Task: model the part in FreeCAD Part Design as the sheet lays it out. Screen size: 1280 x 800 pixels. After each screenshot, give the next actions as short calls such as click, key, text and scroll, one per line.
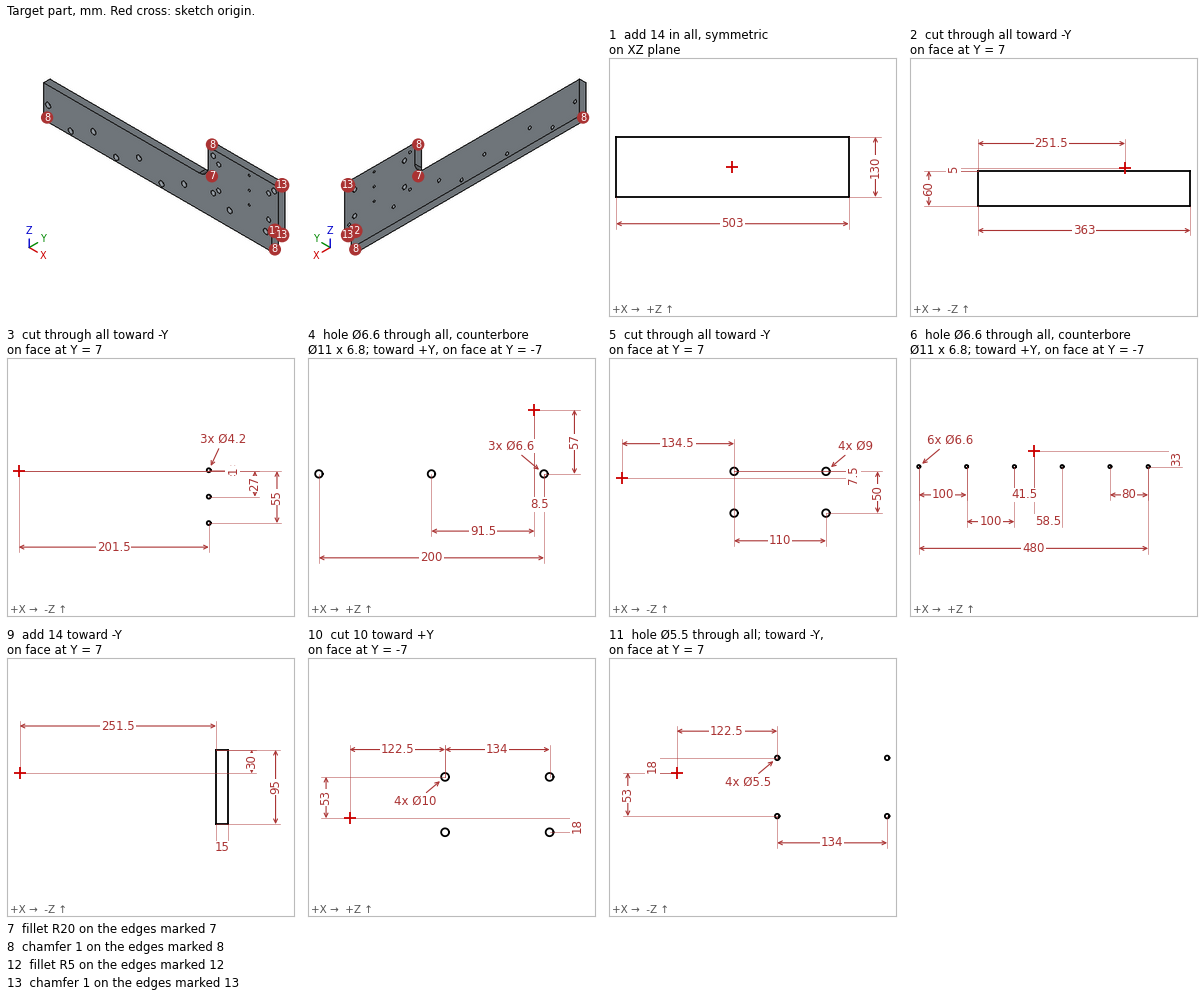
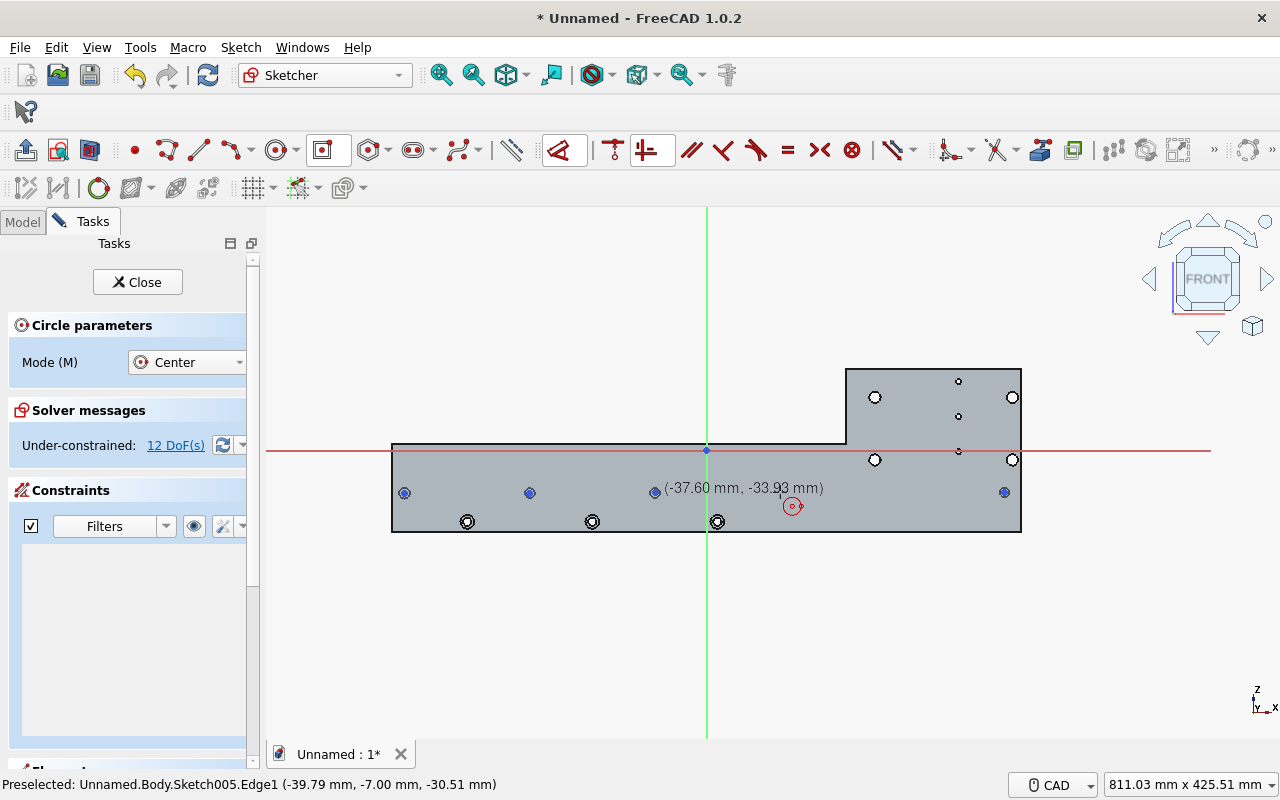
click(780, 492)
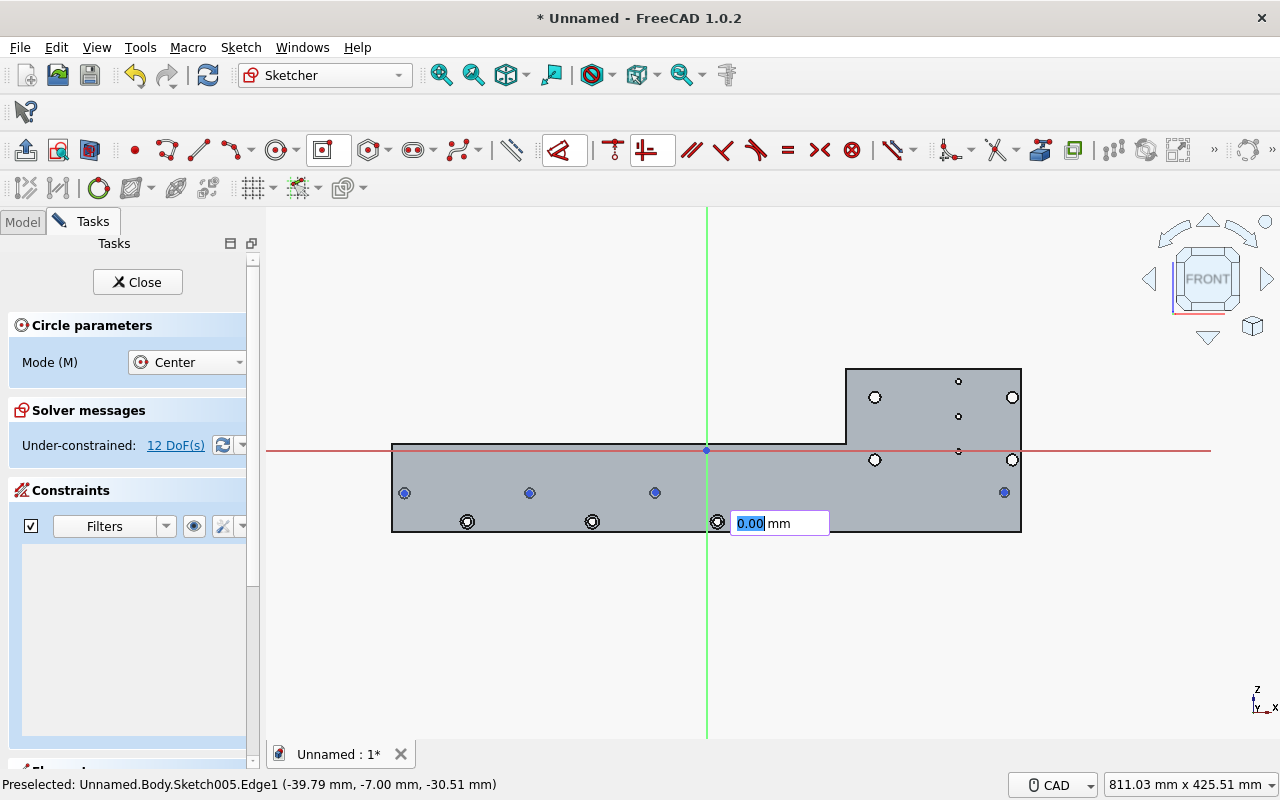
scroll(783, 489, up, 7)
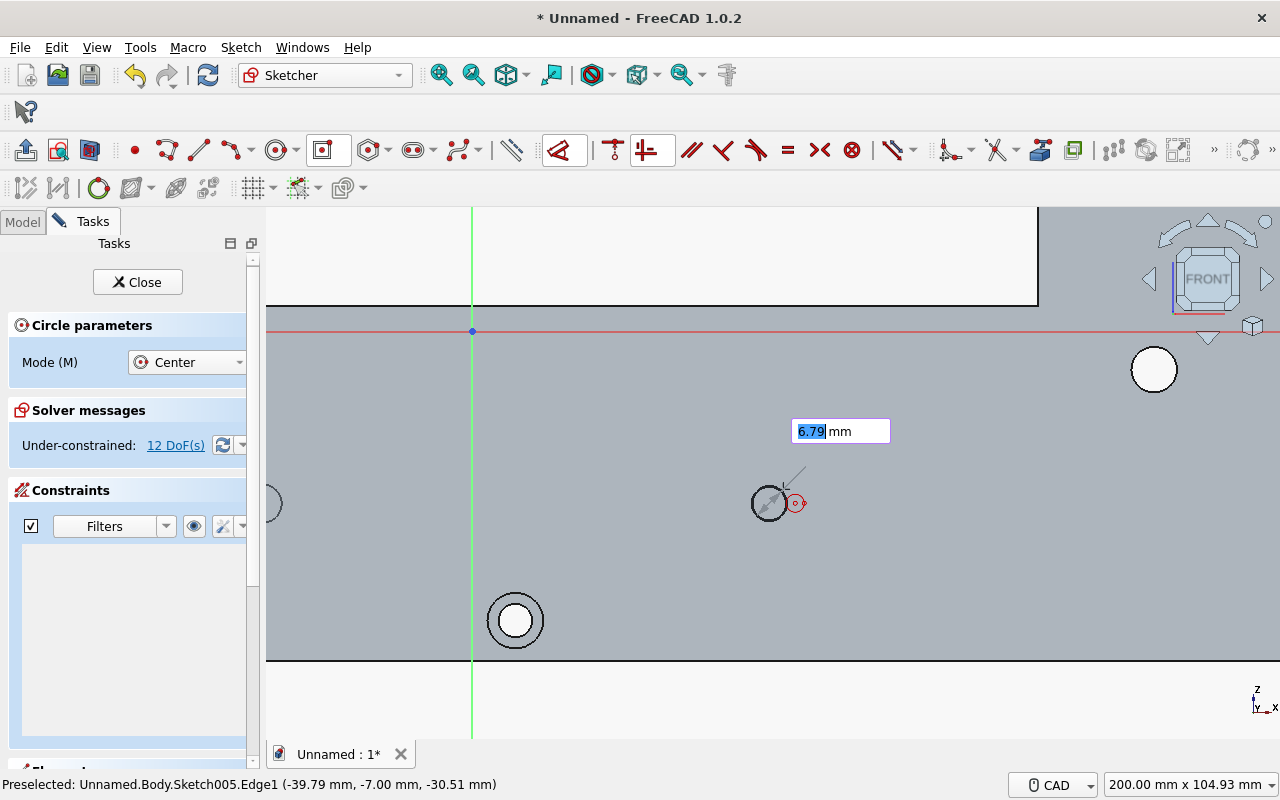
click(781, 487)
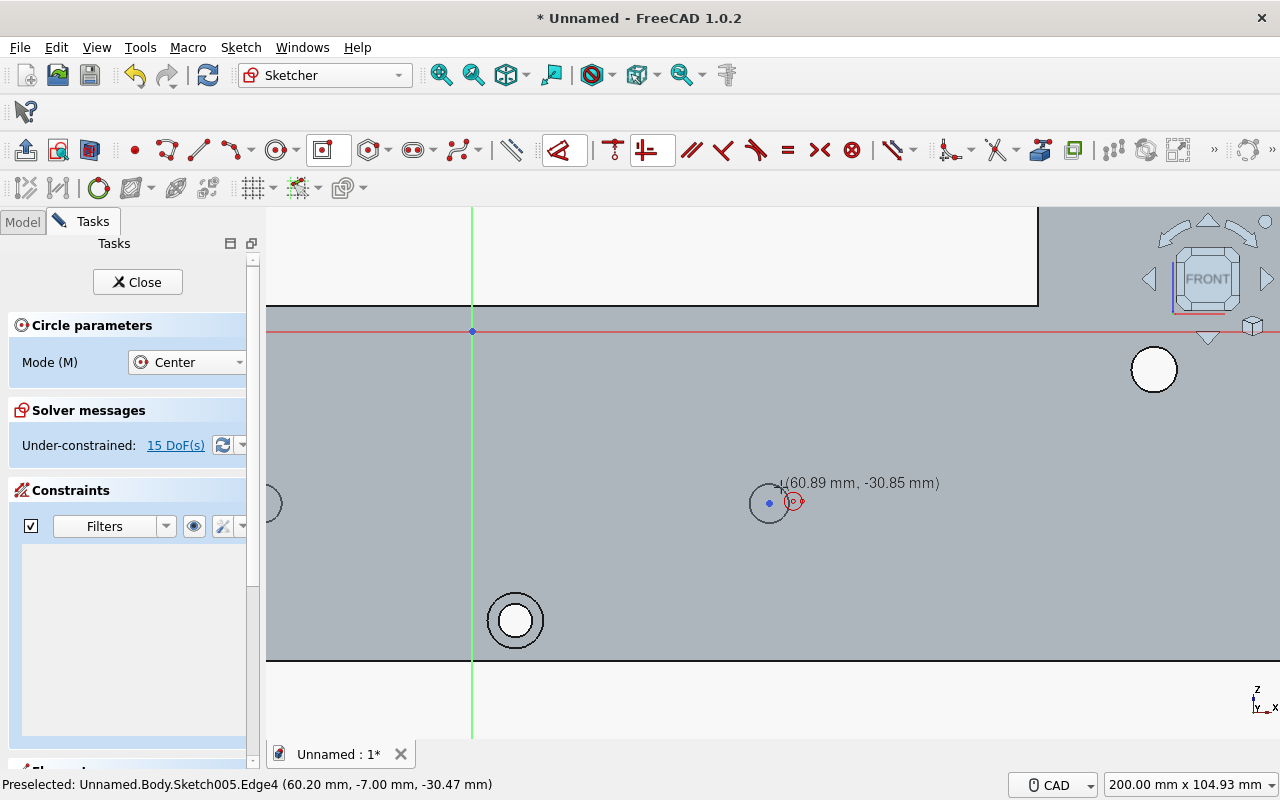
scroll(783, 489, down, 7)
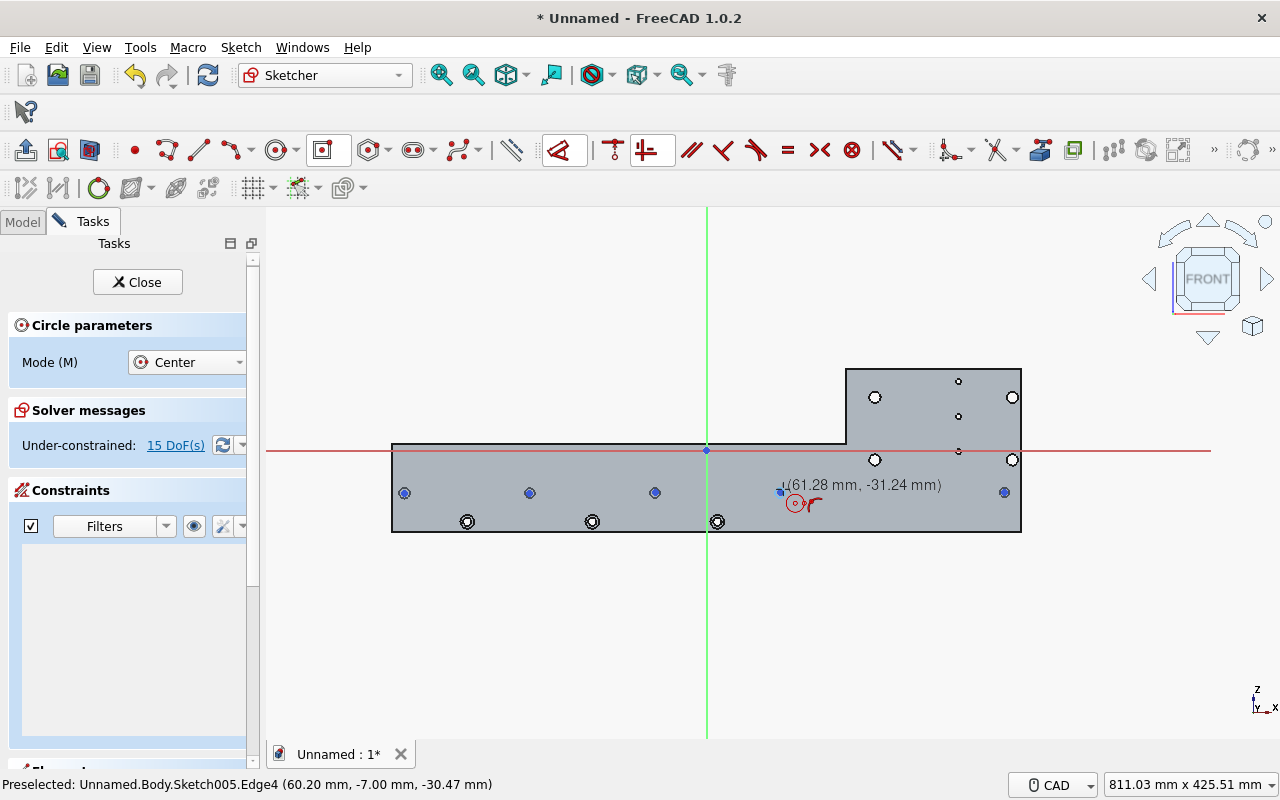
scroll(905, 492, up, 9)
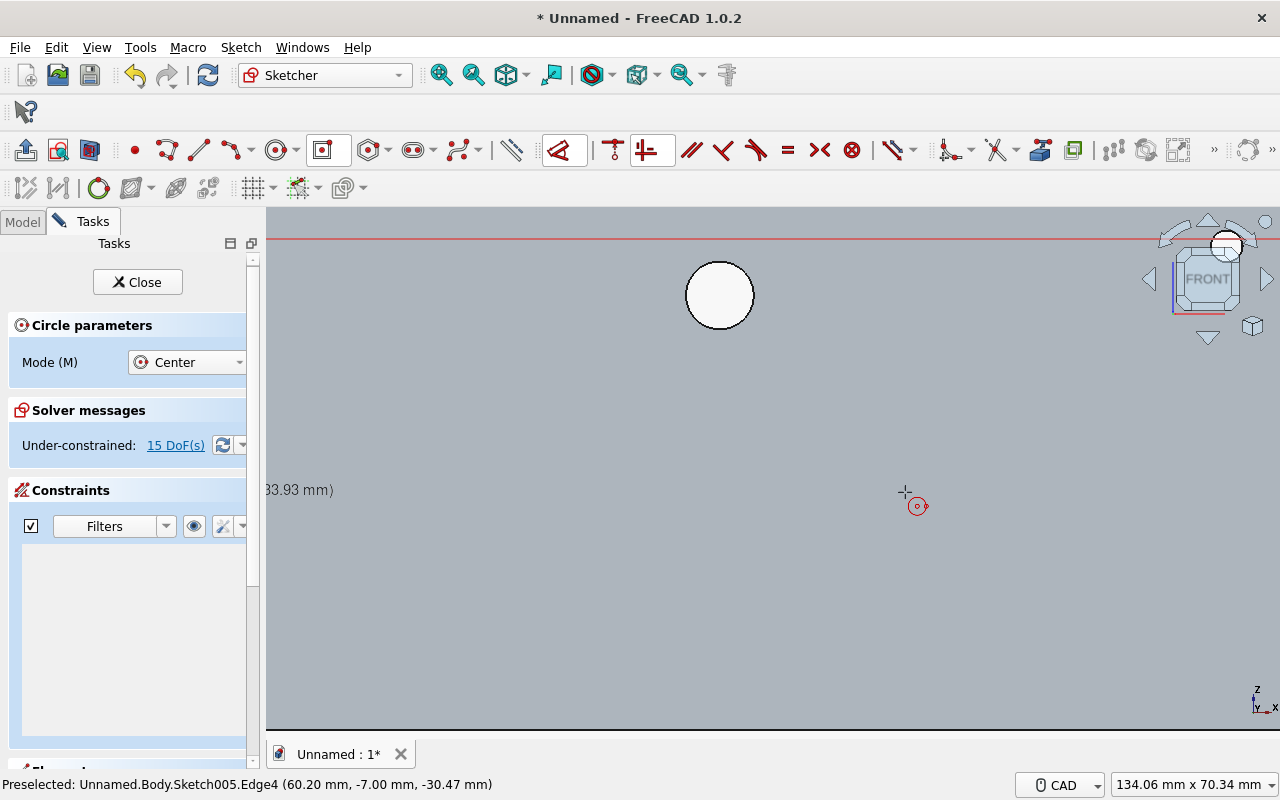
scroll(905, 492, down, 9)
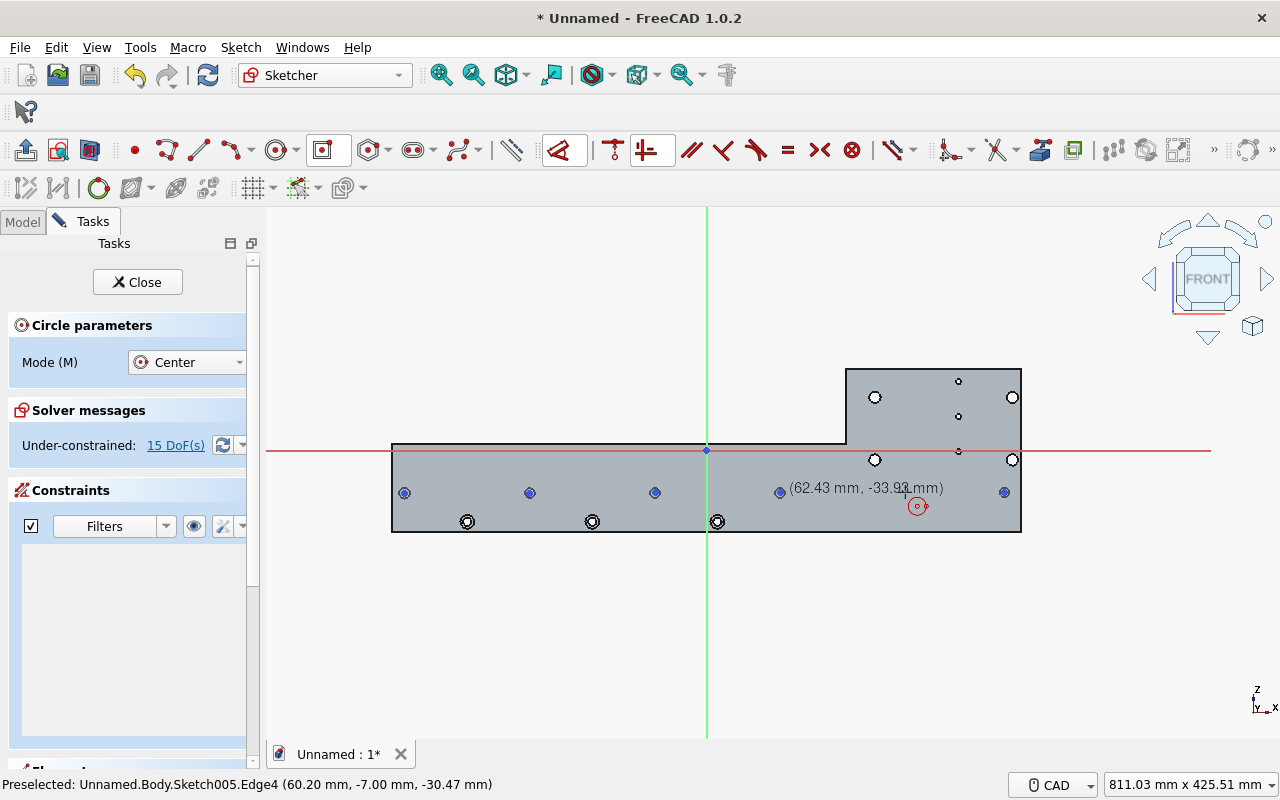
click(905, 492)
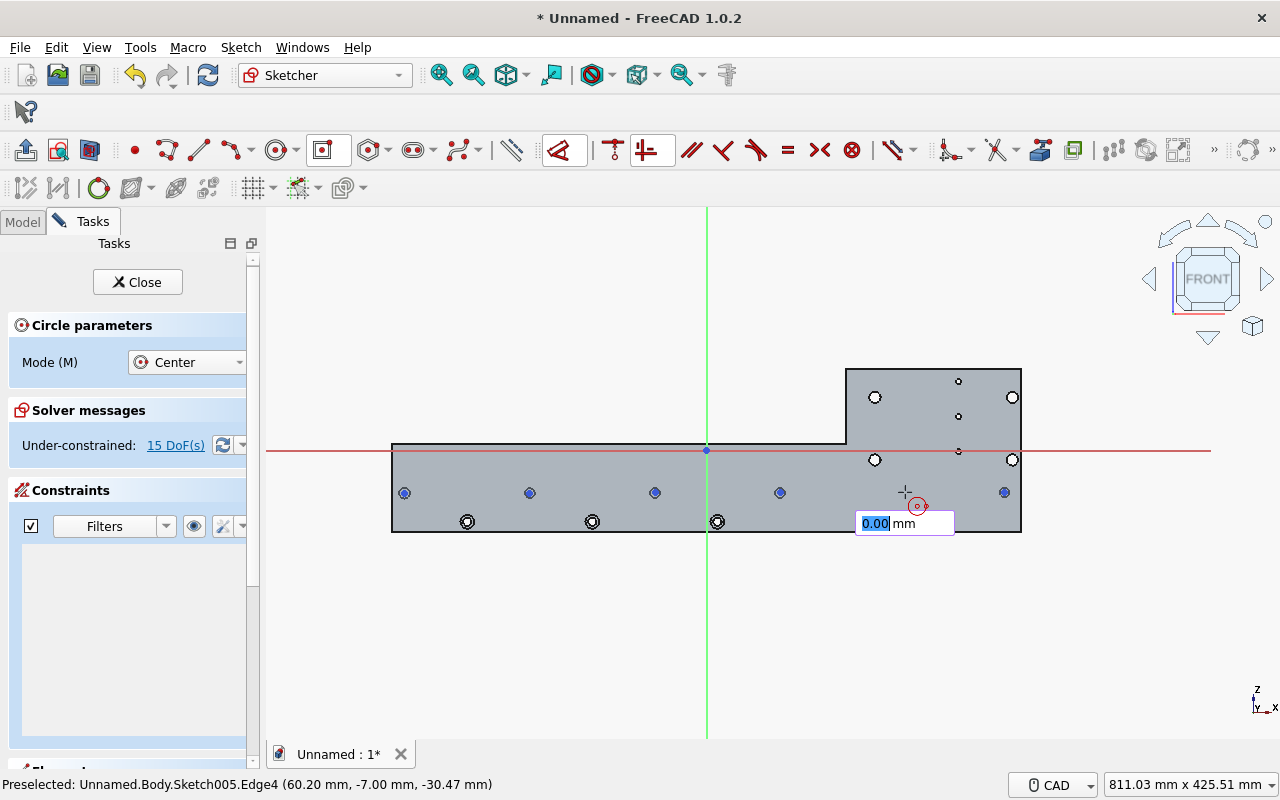
scroll(908, 489, up, 7)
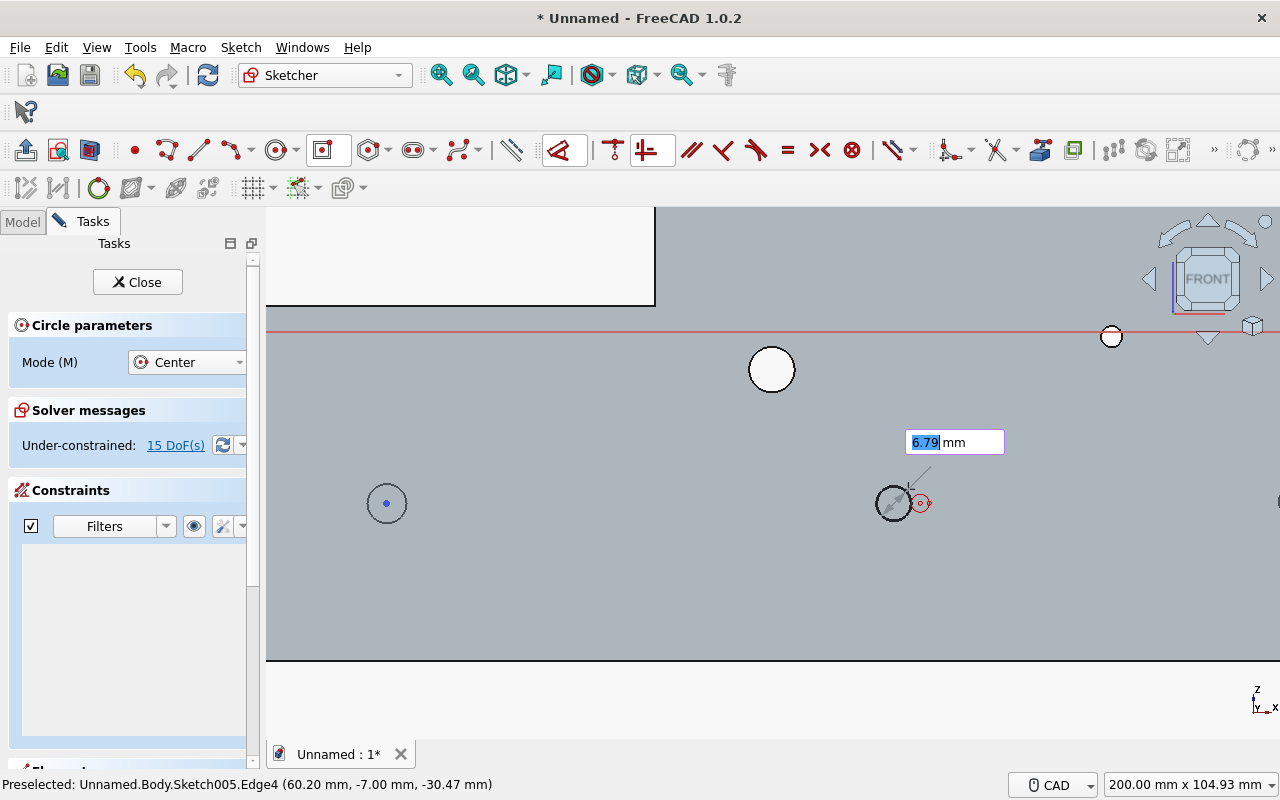
click(905, 487)
key(Escape)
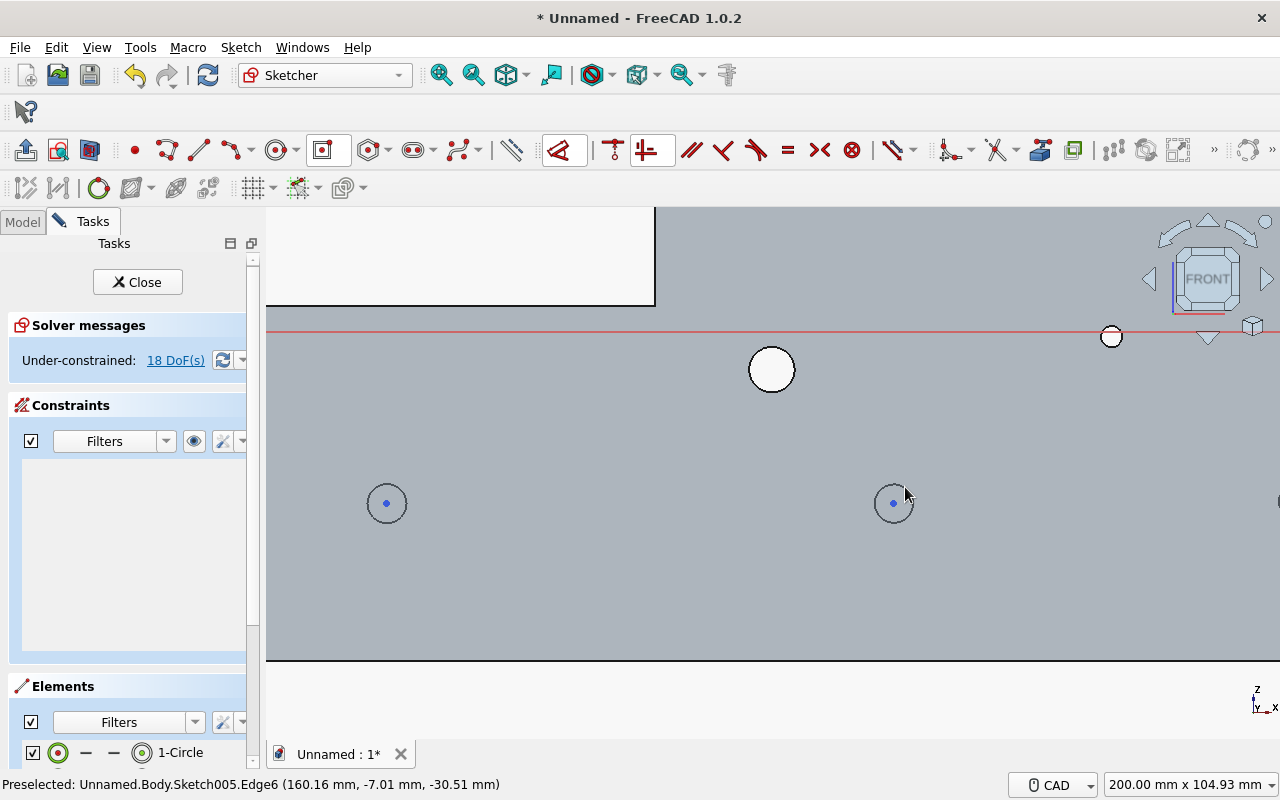
scroll(908, 489, down, 7)